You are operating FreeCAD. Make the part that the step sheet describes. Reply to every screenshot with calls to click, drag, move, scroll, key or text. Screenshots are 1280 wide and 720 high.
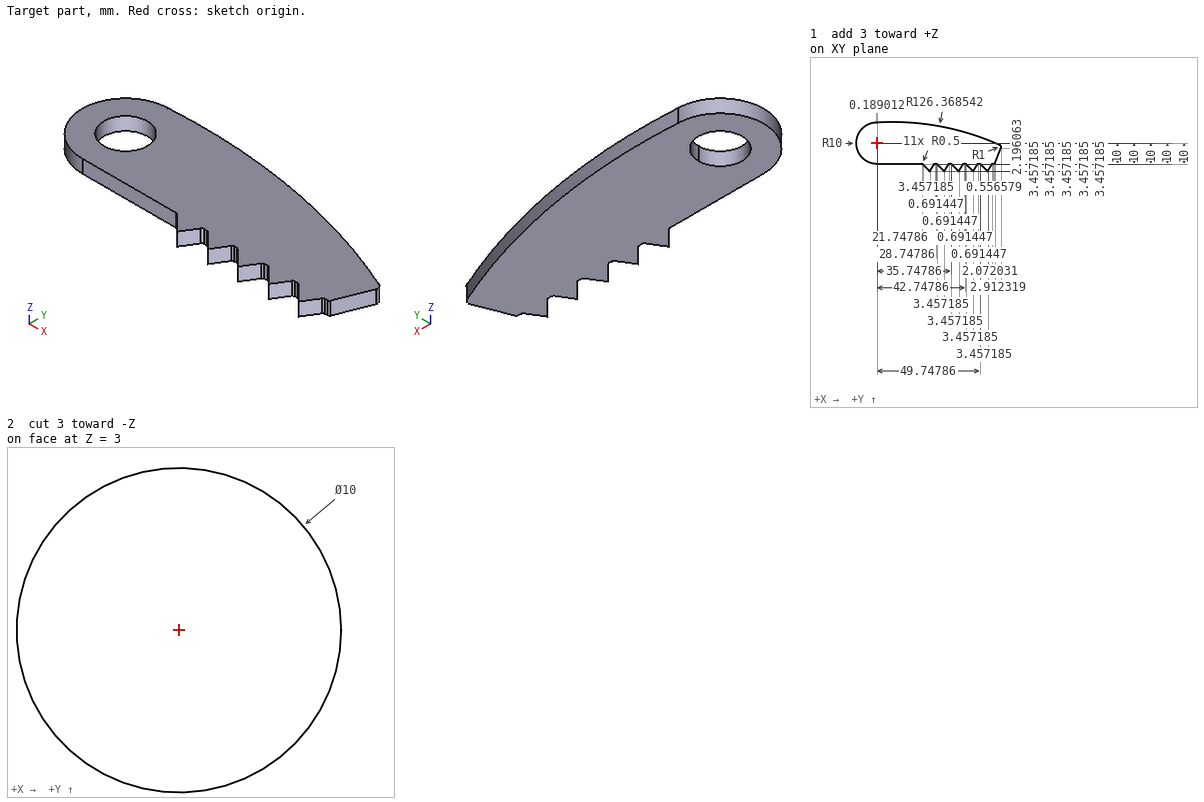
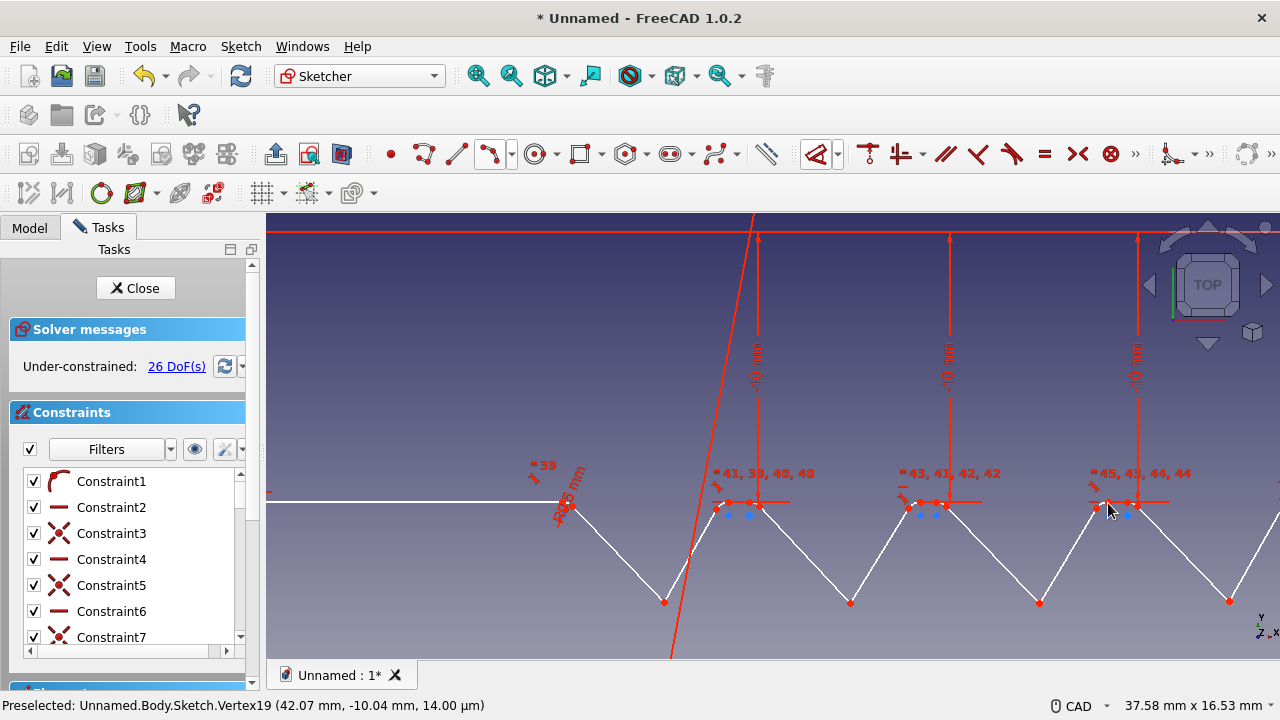
scroll(729, 503, down, 6)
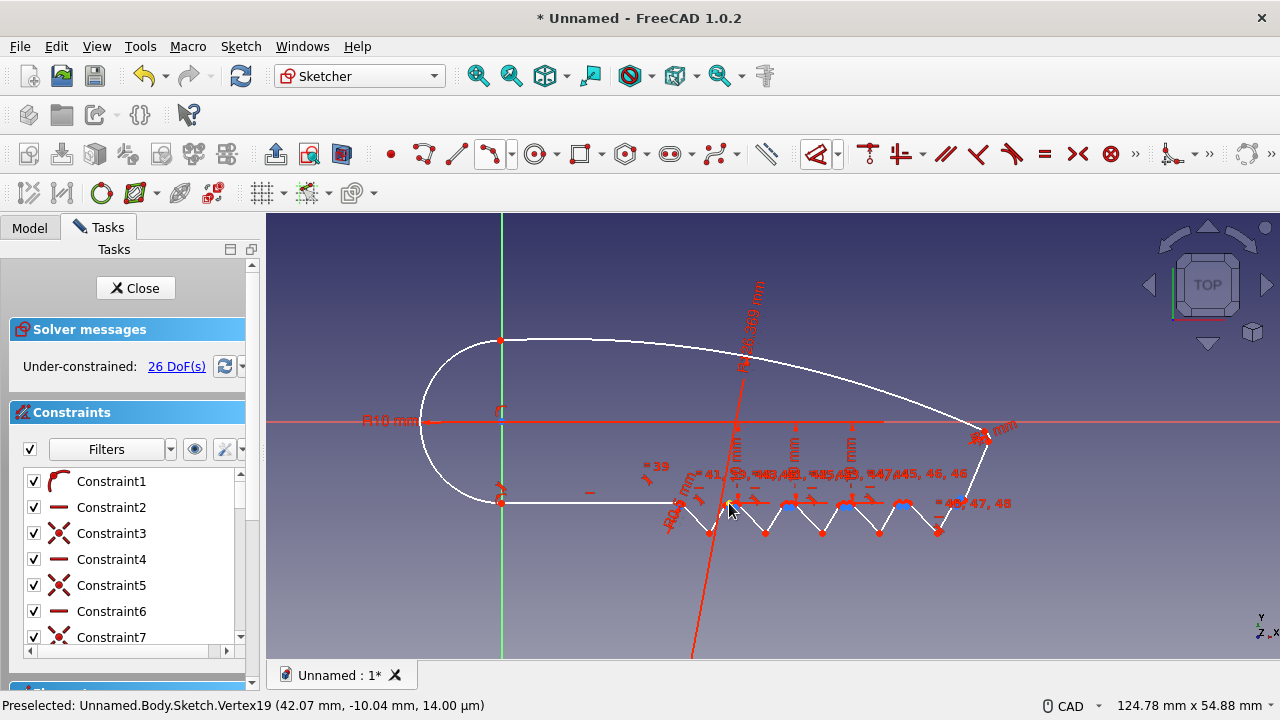
scroll(900, 502, up, 6)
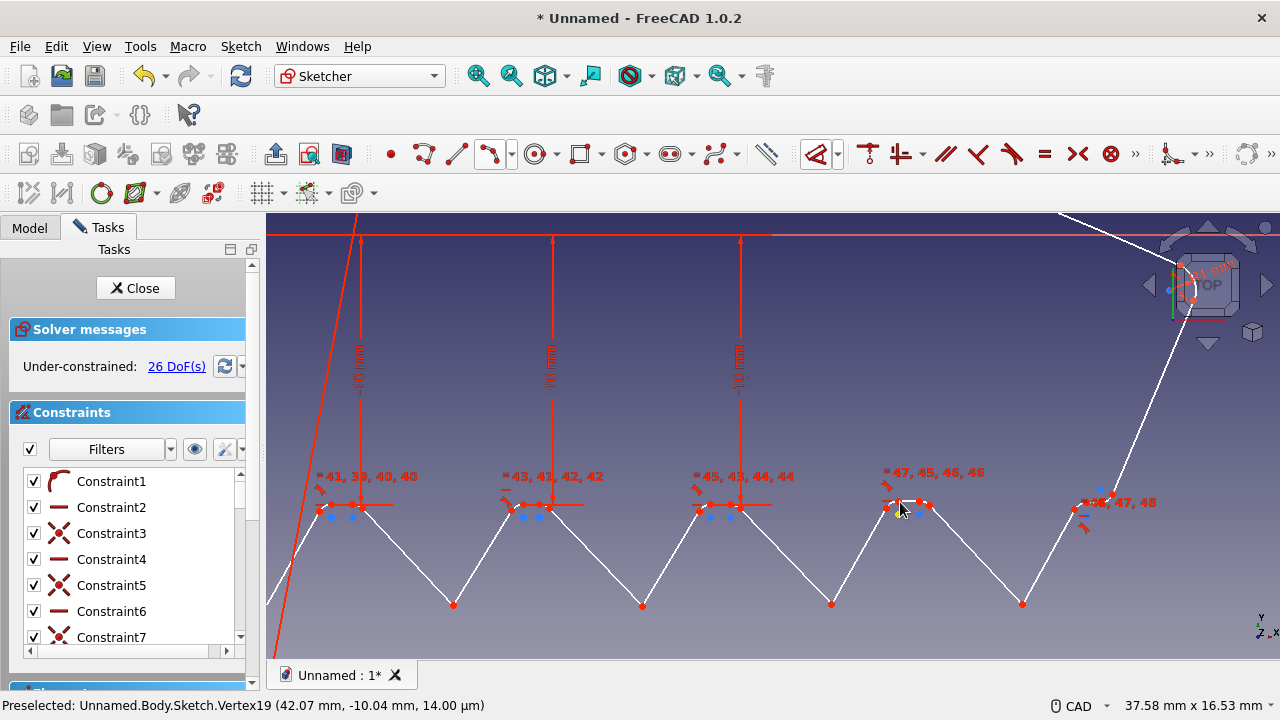
click(898, 501)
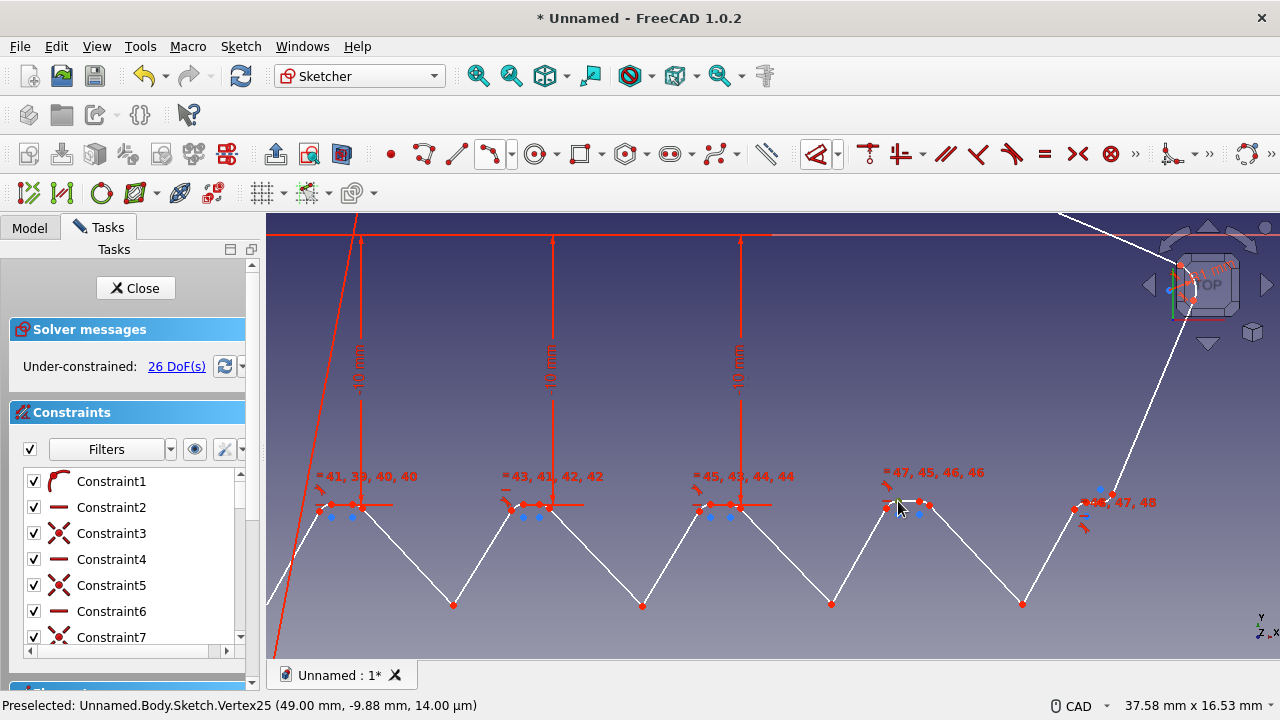
click(838, 154)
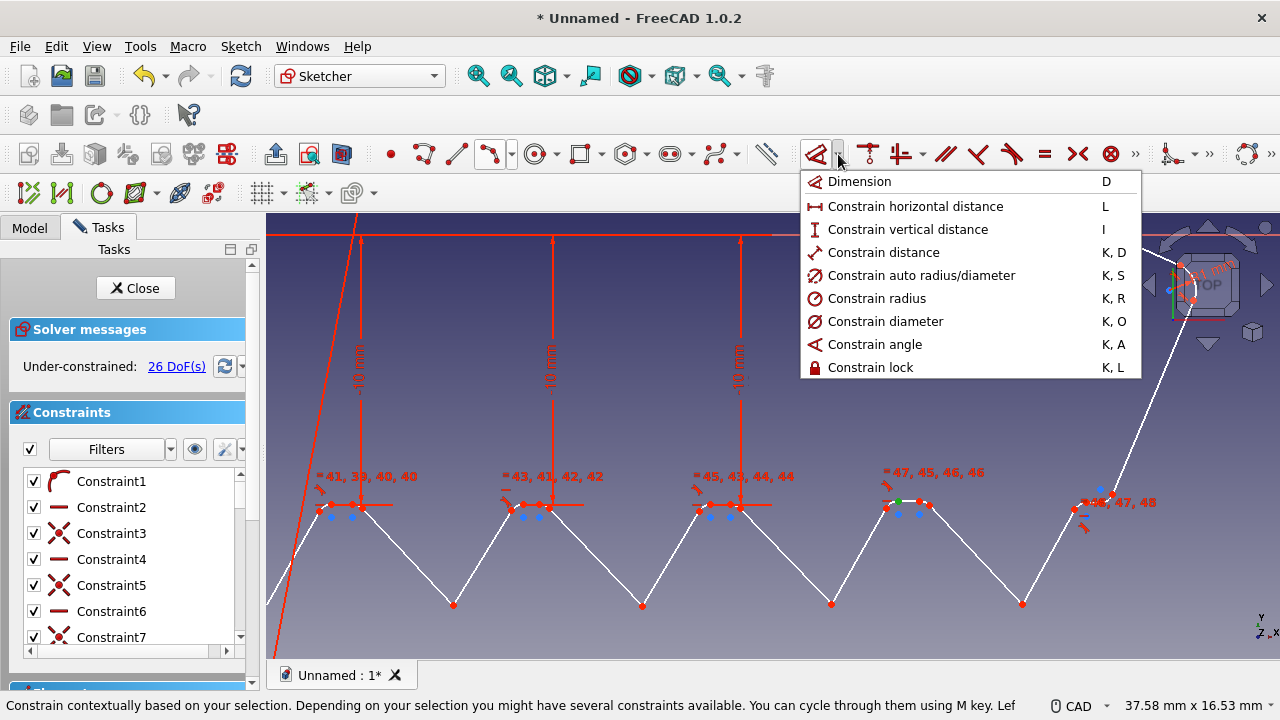
click(971, 230)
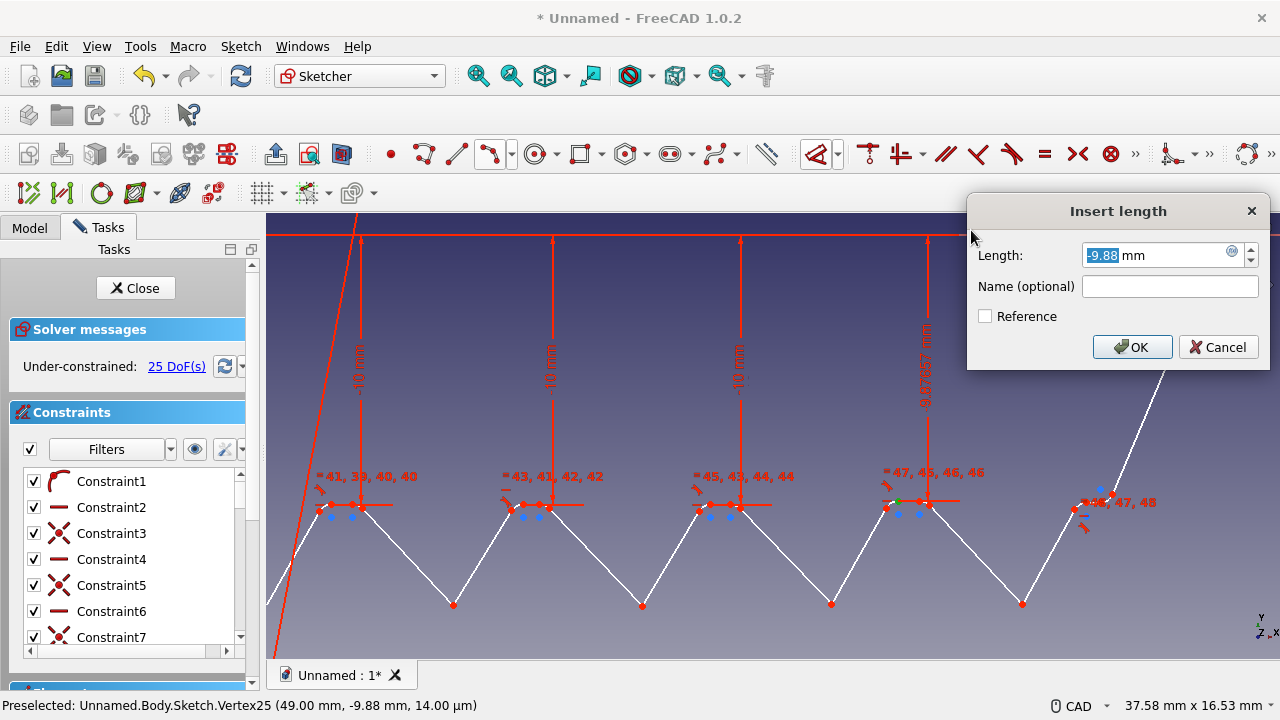
text(-10)
key(Return)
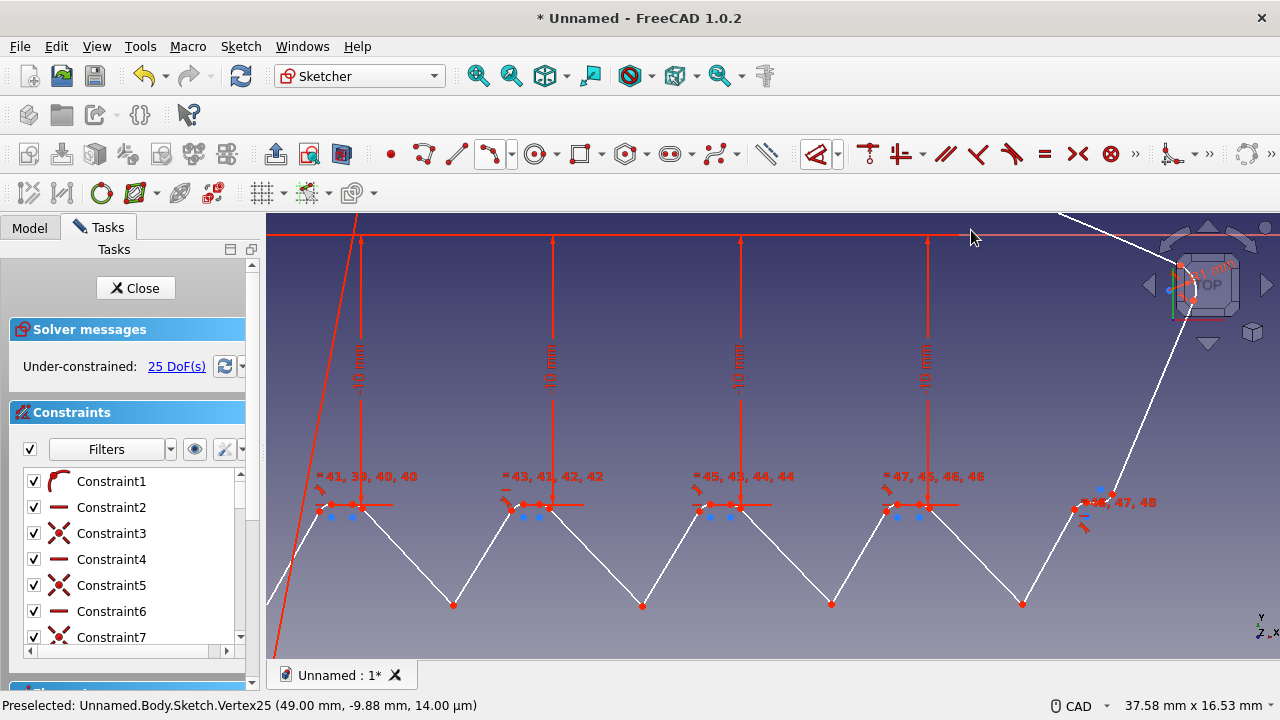
scroll(1087, 503, up, 4)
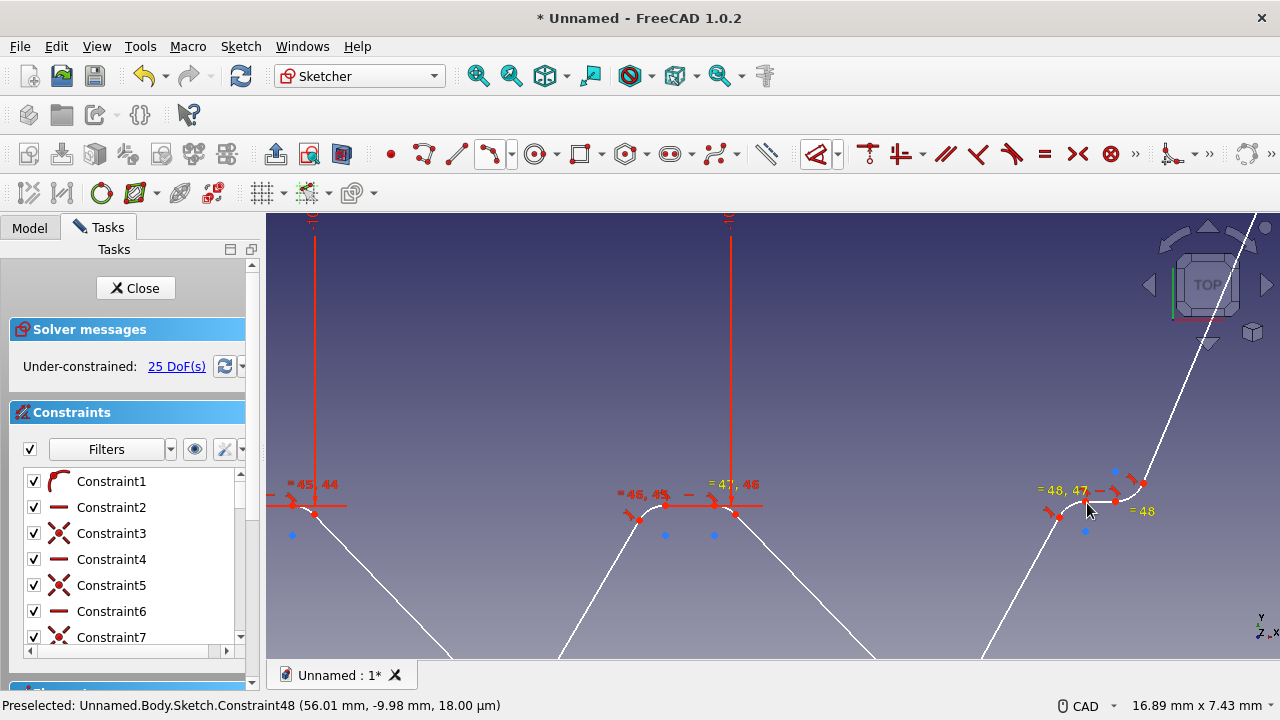
click(1086, 502)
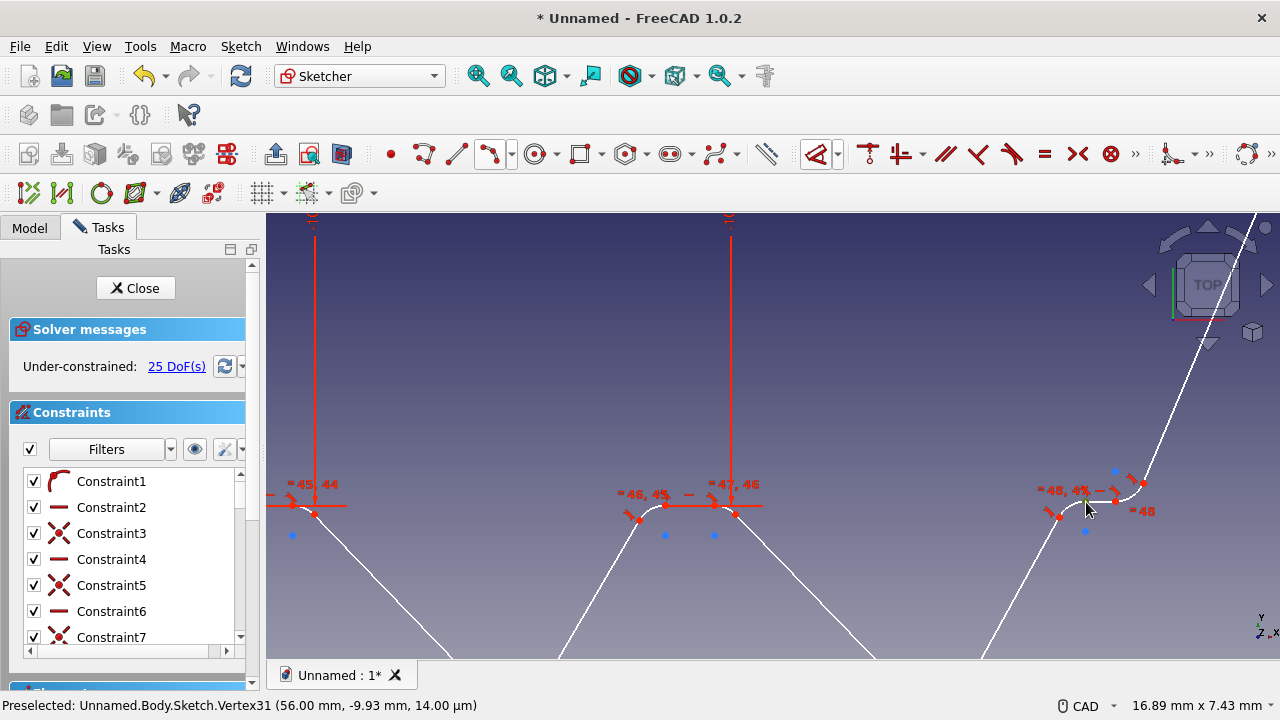
key(i)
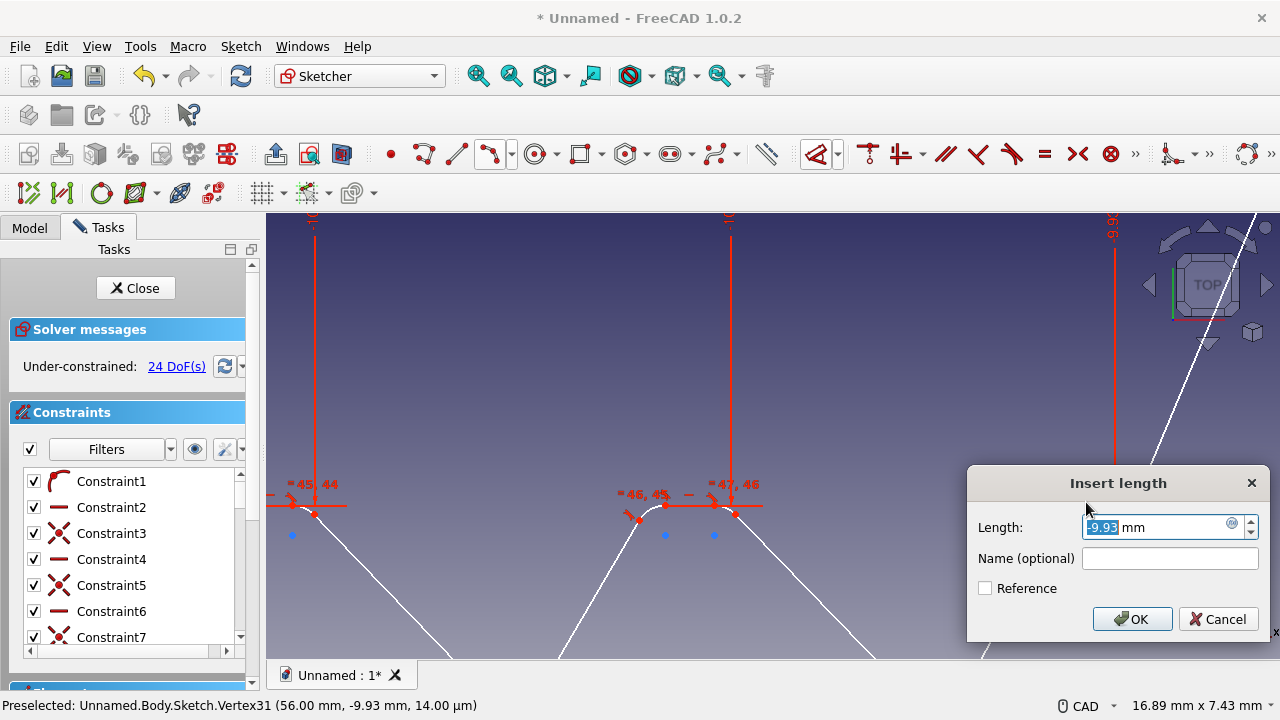
text(-10)
key(Return)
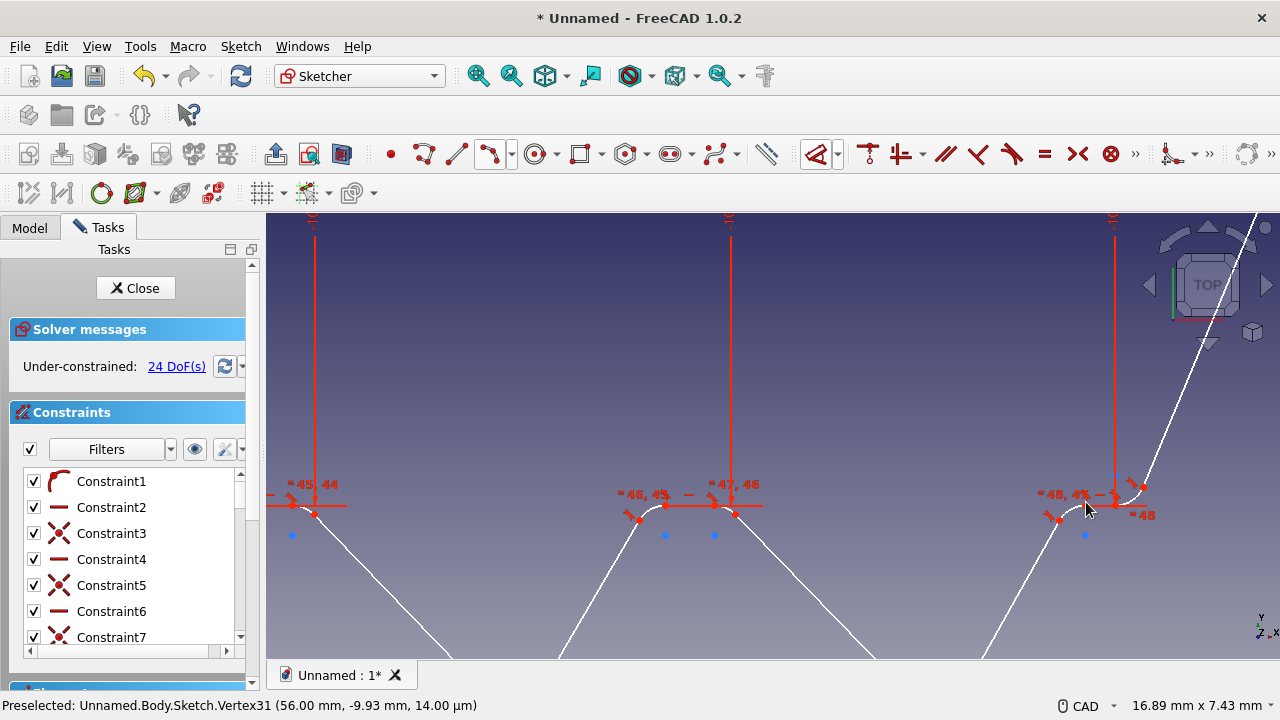
scroll(936, 502, down, 10)